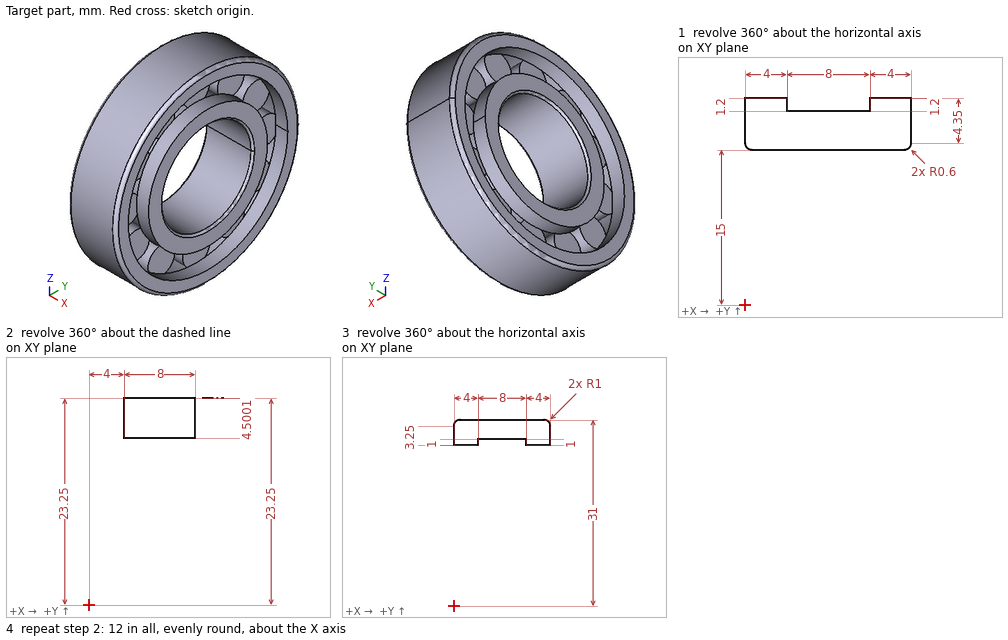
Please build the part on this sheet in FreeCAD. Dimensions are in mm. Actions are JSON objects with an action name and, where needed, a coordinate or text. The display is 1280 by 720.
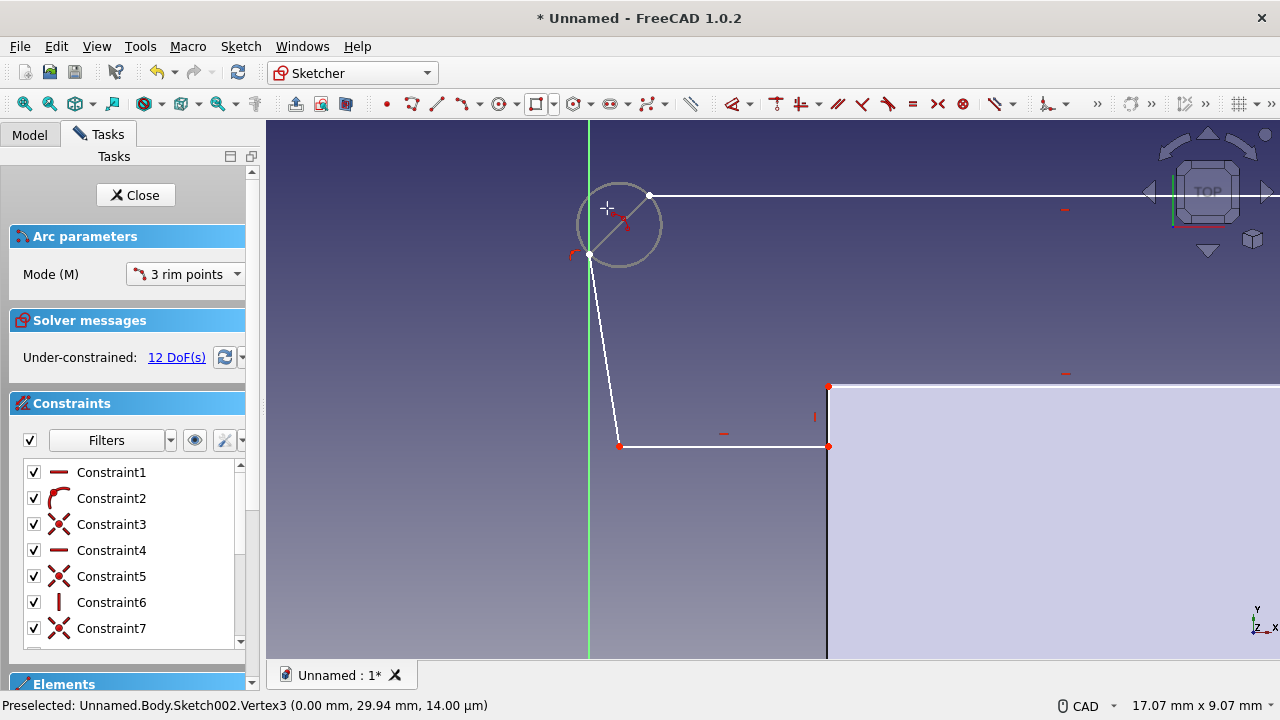
{"action": "left_click", "coordinate": [607, 208]}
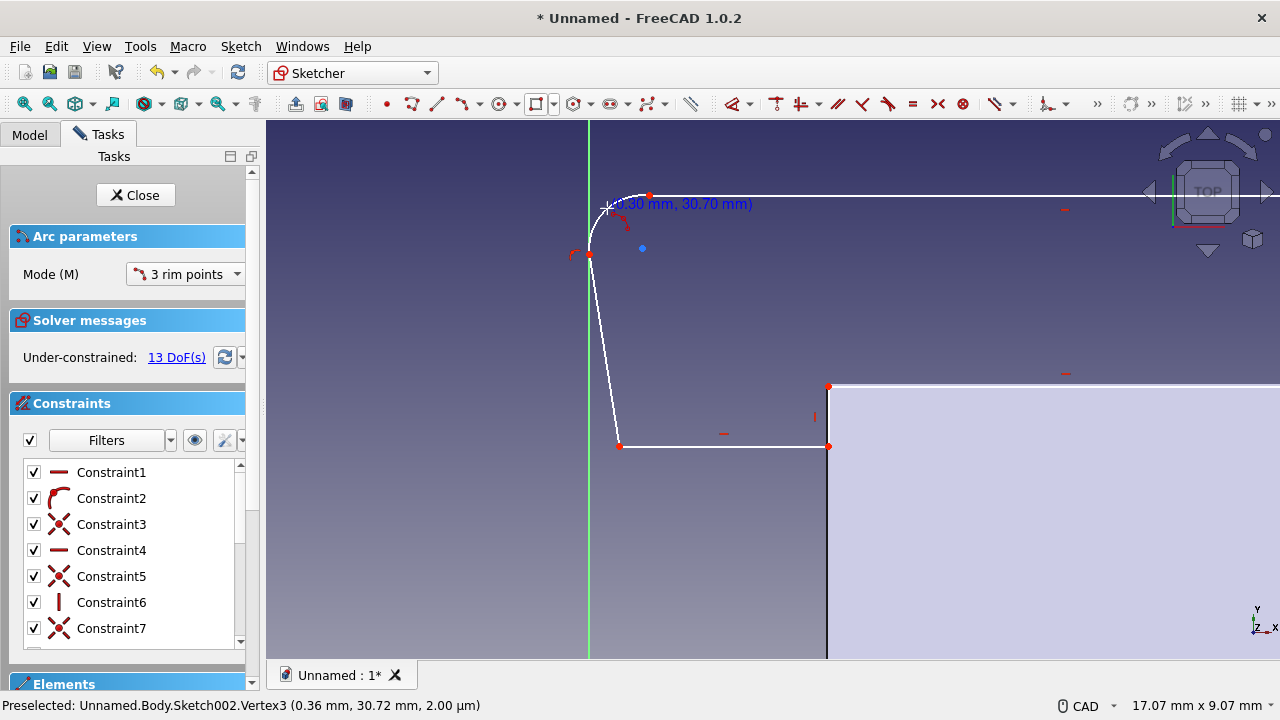
{"action": "scroll", "coordinate": [613, 207], "scroll_direction": "down", "scroll_amount": 8}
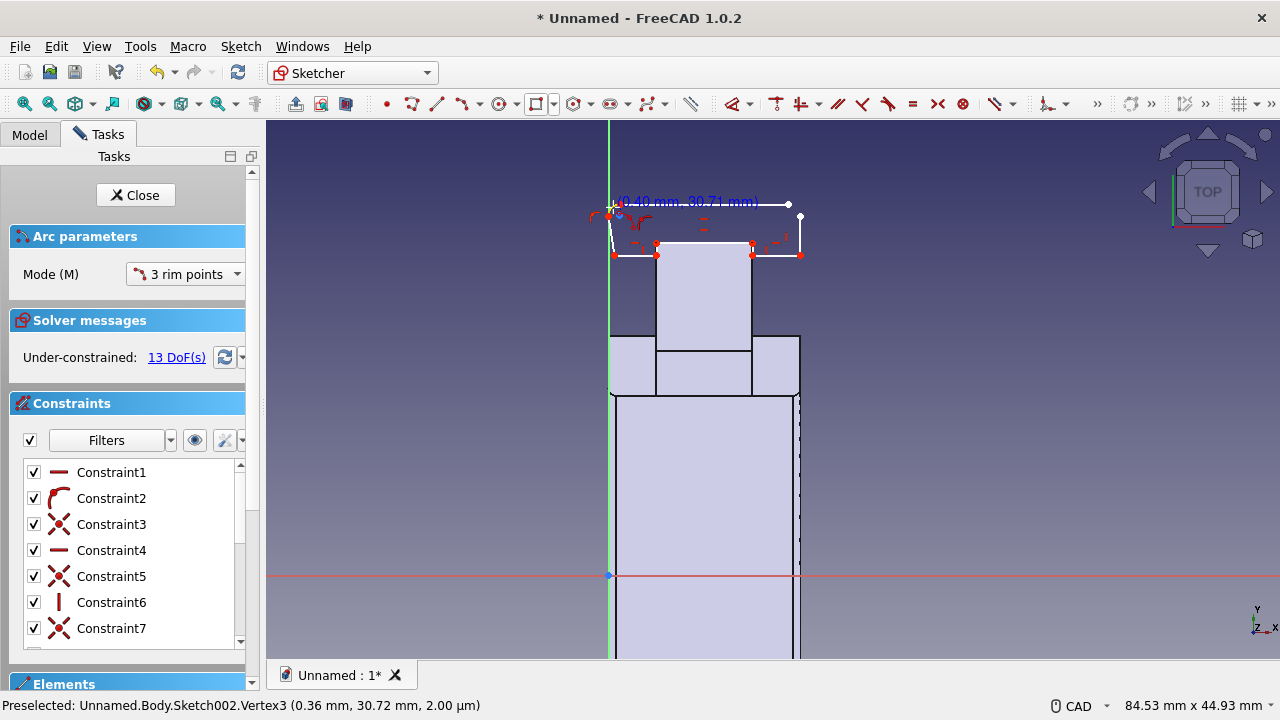
{"action": "left_click", "coordinate": [800, 217]}
{"action": "left_click", "coordinate": [789, 205]}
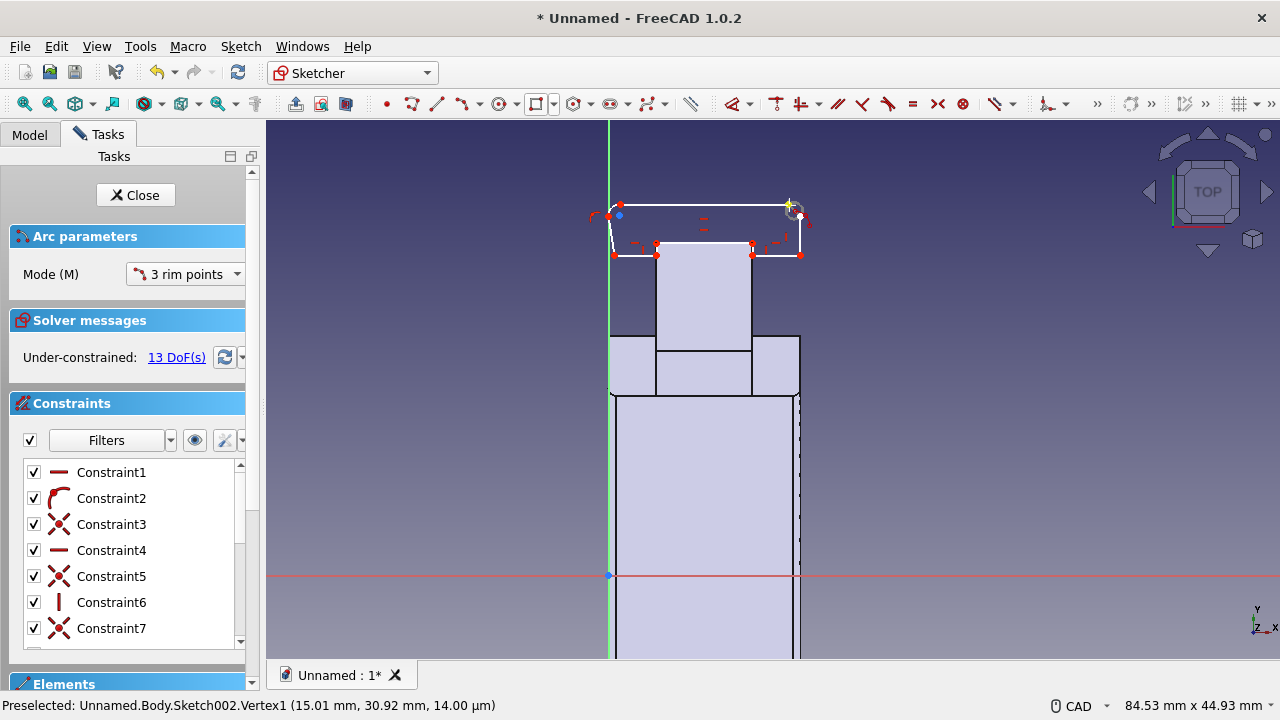
{"action": "scroll", "coordinate": [797, 207], "scroll_direction": "up", "scroll_amount": 8}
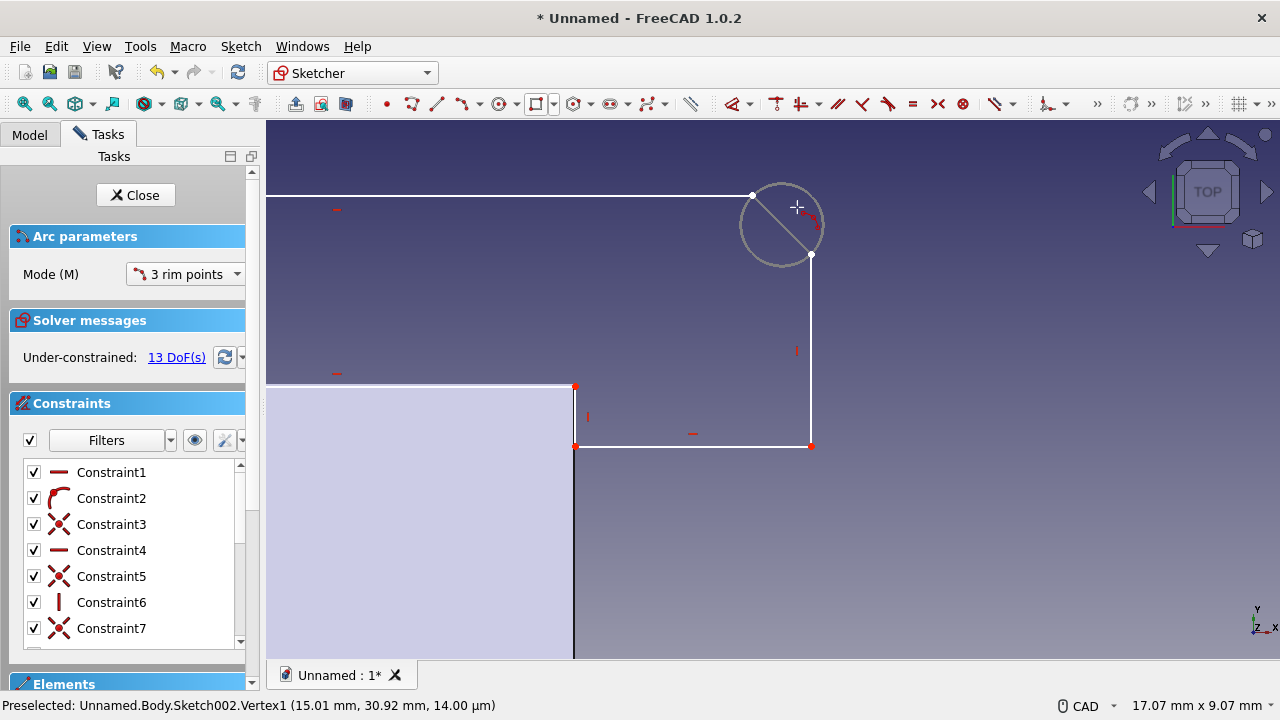
{"action": "left_click", "coordinate": [795, 208]}
{"action": "key", "text": "Escape"}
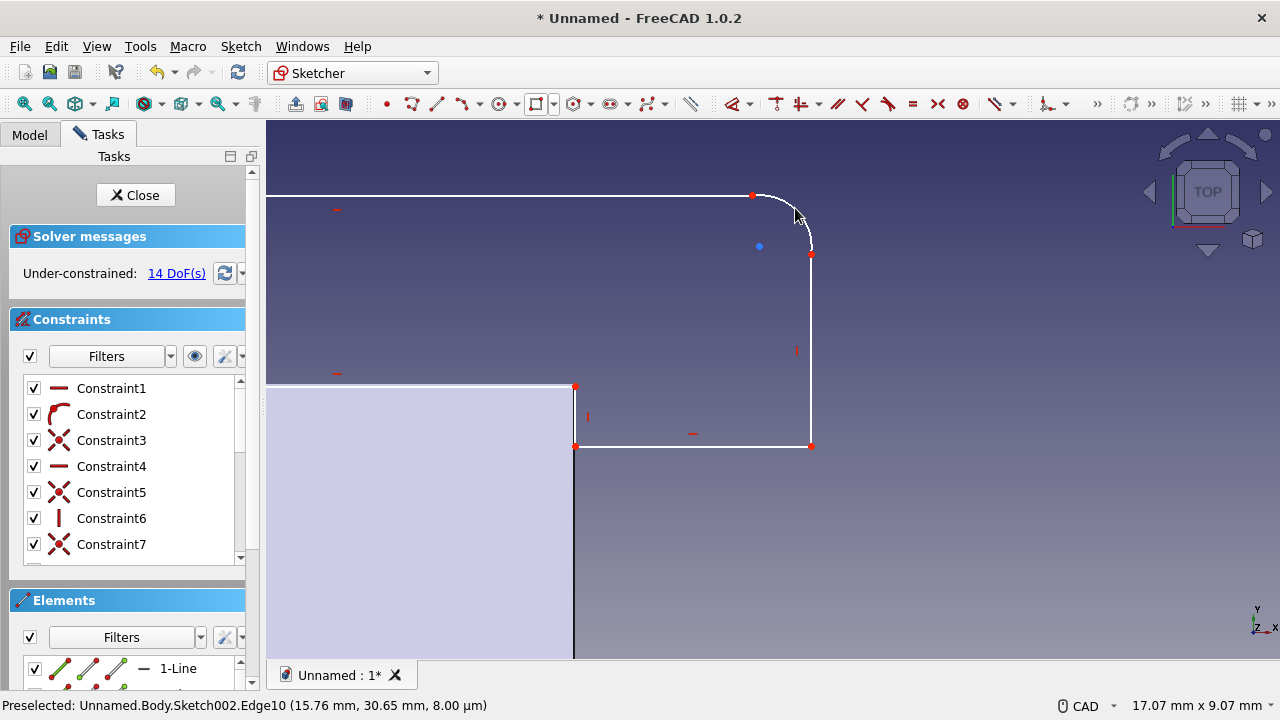
{"action": "scroll", "coordinate": [798, 207], "scroll_direction": "down", "scroll_amount": 8}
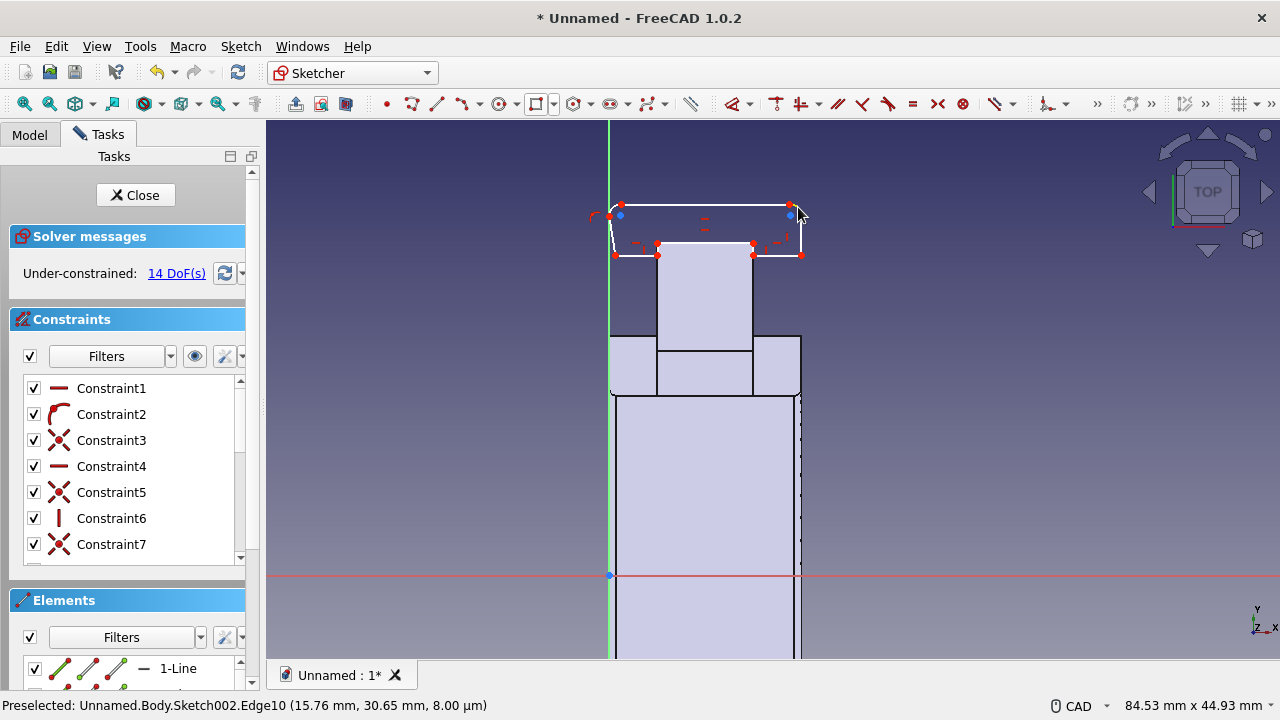
{"action": "left_click", "coordinate": [739, 205]}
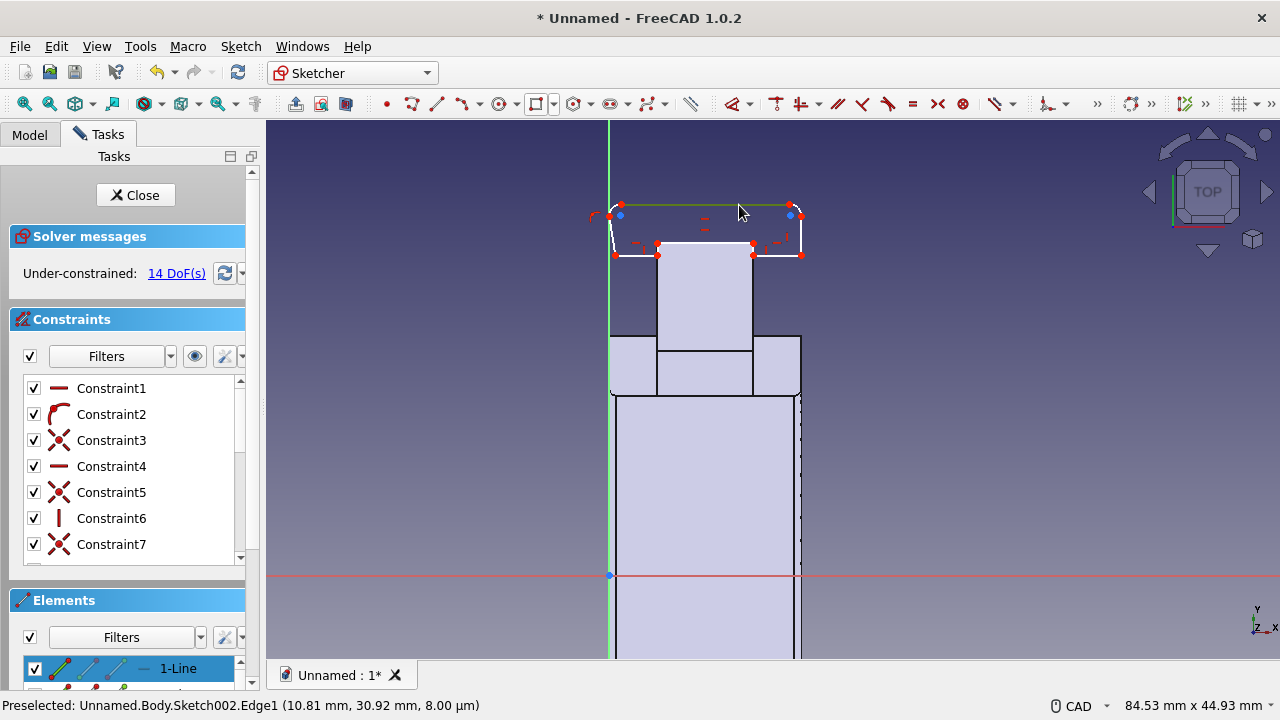
{"action": "scroll", "coordinate": [613, 208], "scroll_direction": "up", "scroll_amount": 2}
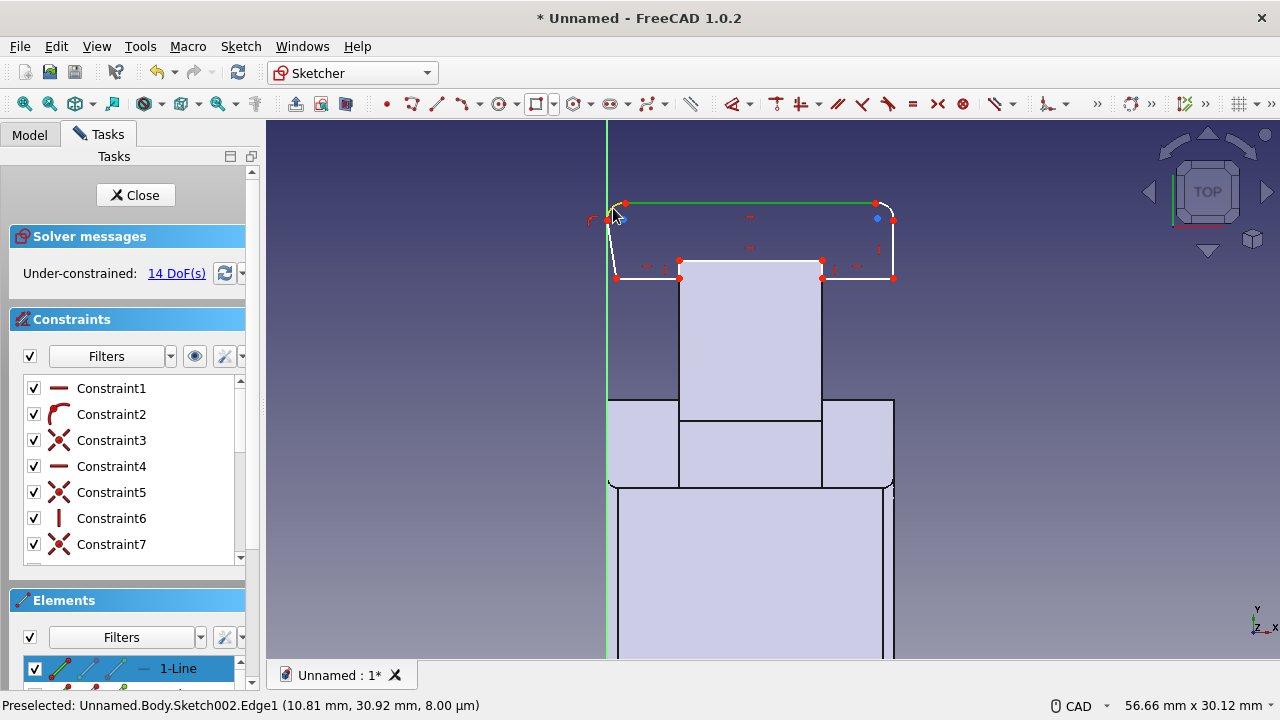
{"action": "left_click", "coordinate": [612, 208]}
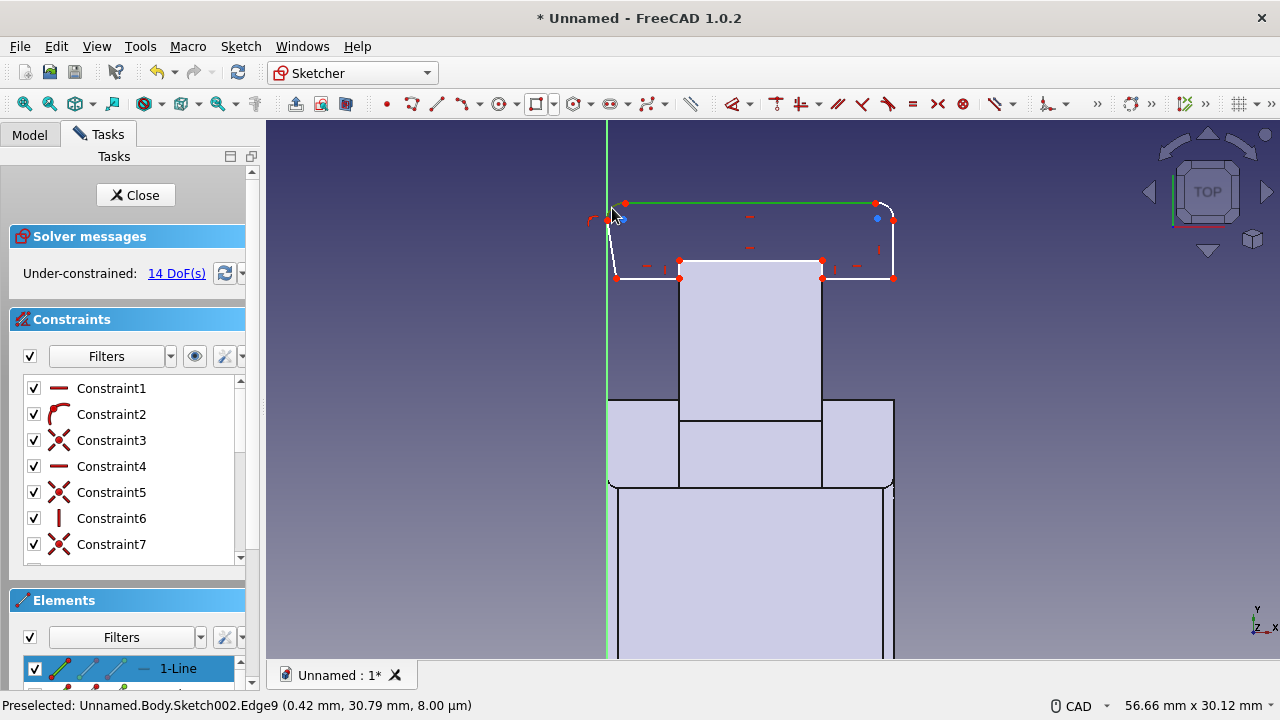
{"action": "left_click", "coordinate": [888, 104]}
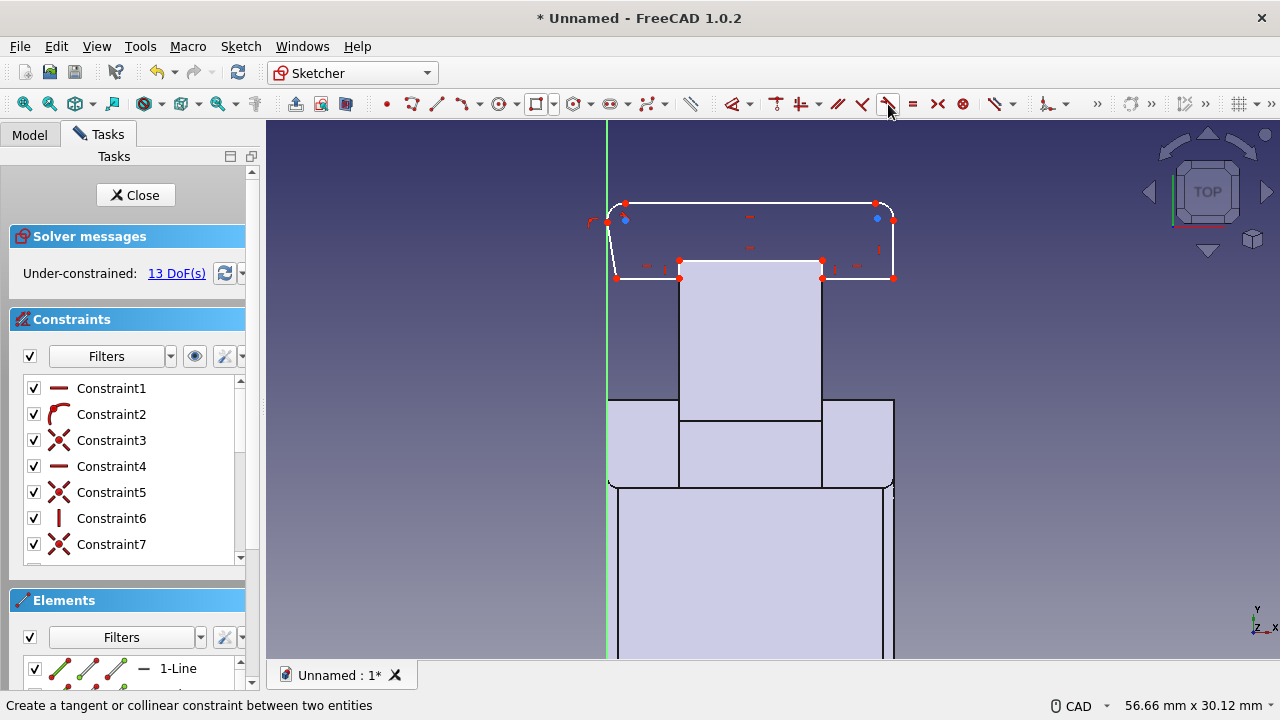
{"action": "left_click", "coordinate": [801, 203]}